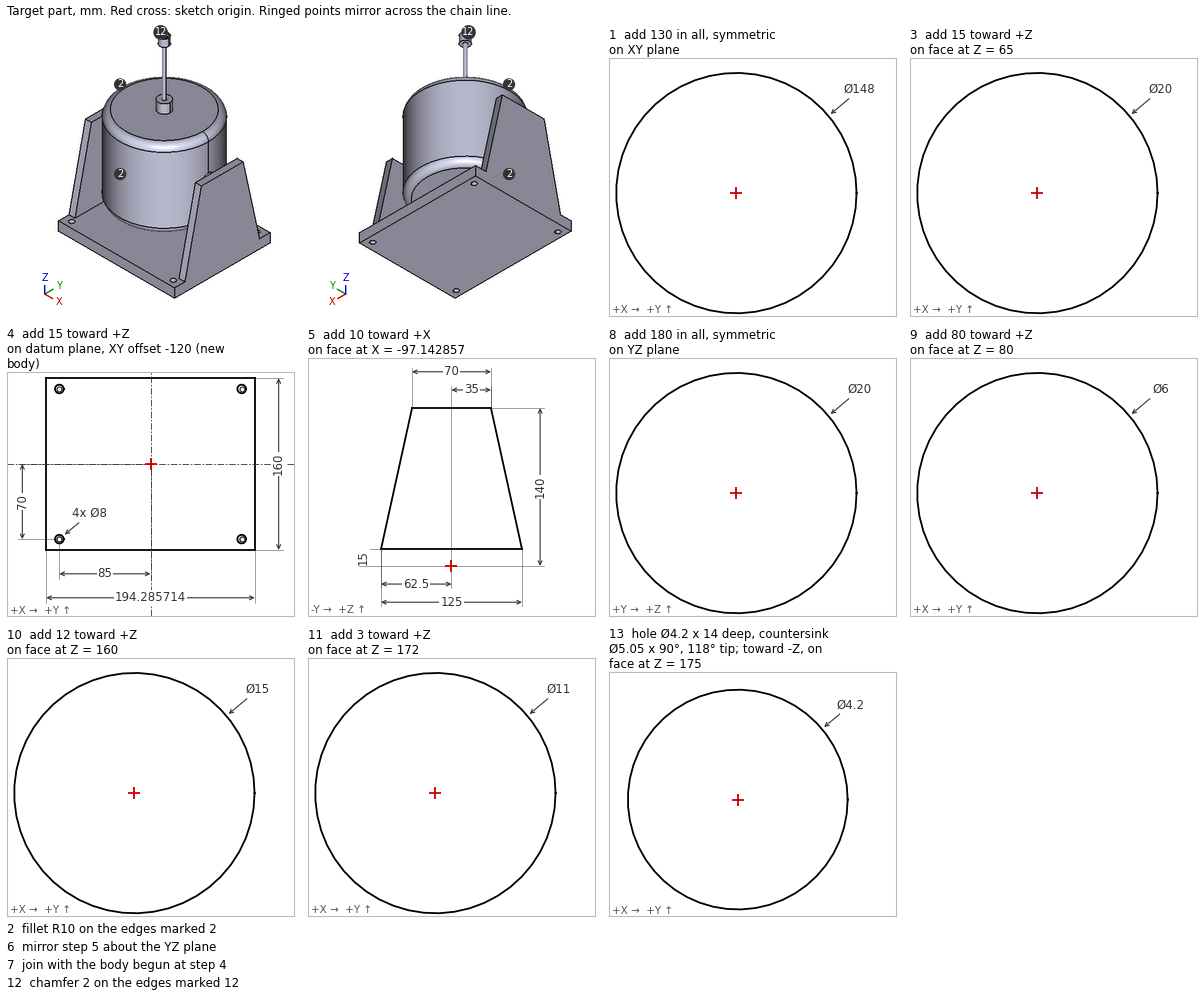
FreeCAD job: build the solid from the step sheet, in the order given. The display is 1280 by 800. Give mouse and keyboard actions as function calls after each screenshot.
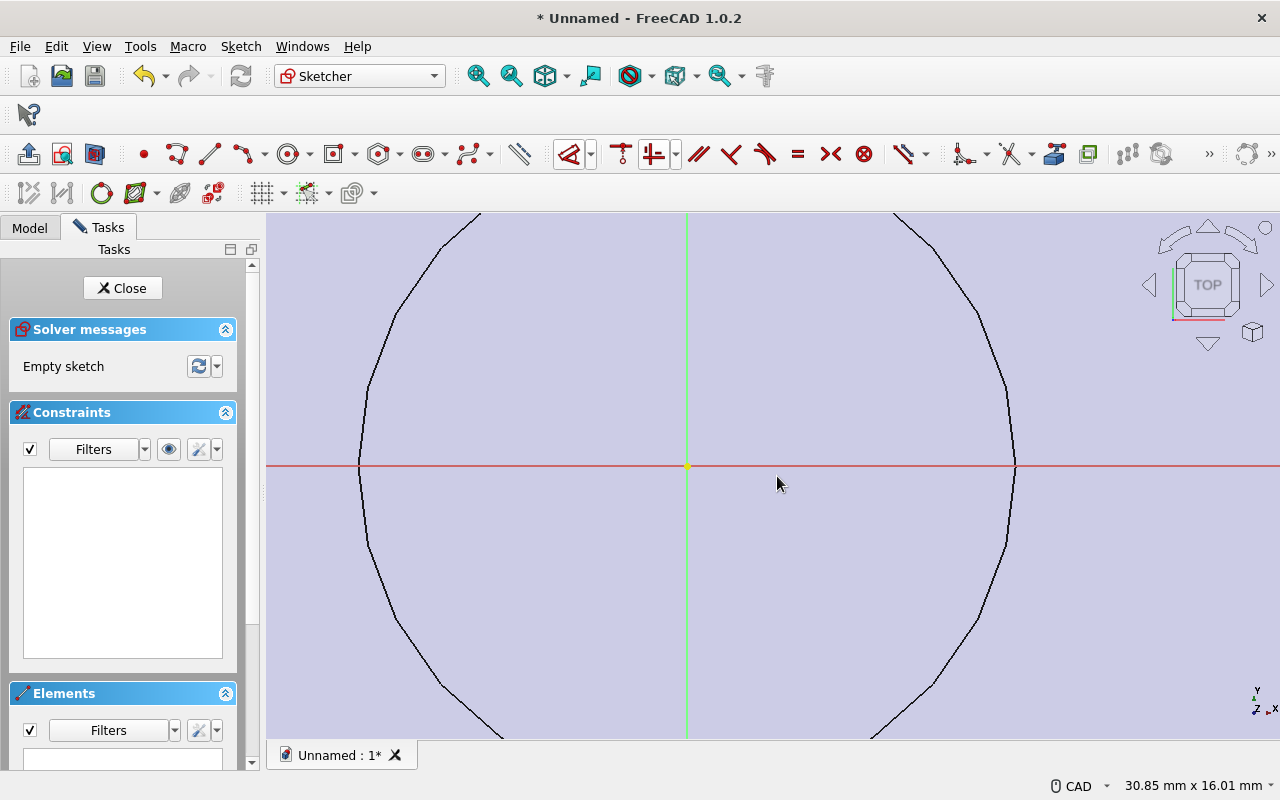
scroll(666, 455, up, 3)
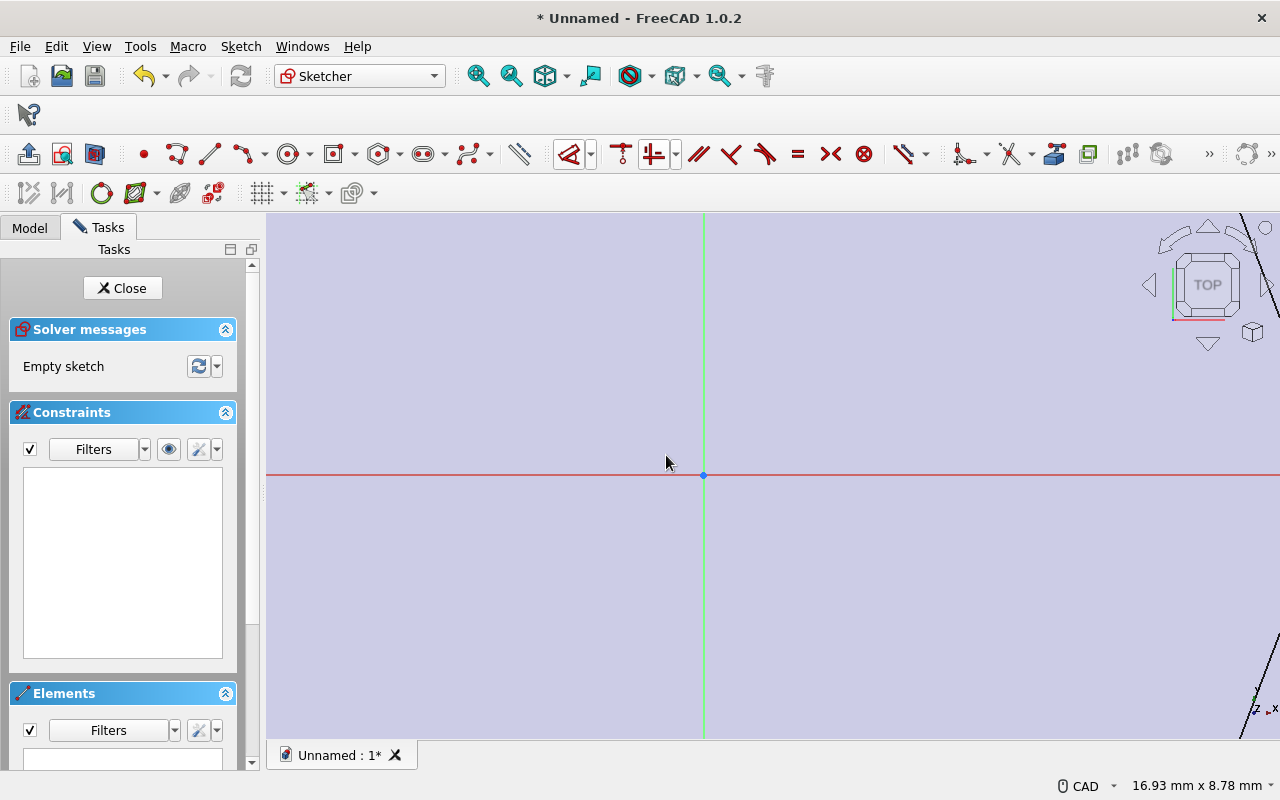
key(g)
key(c)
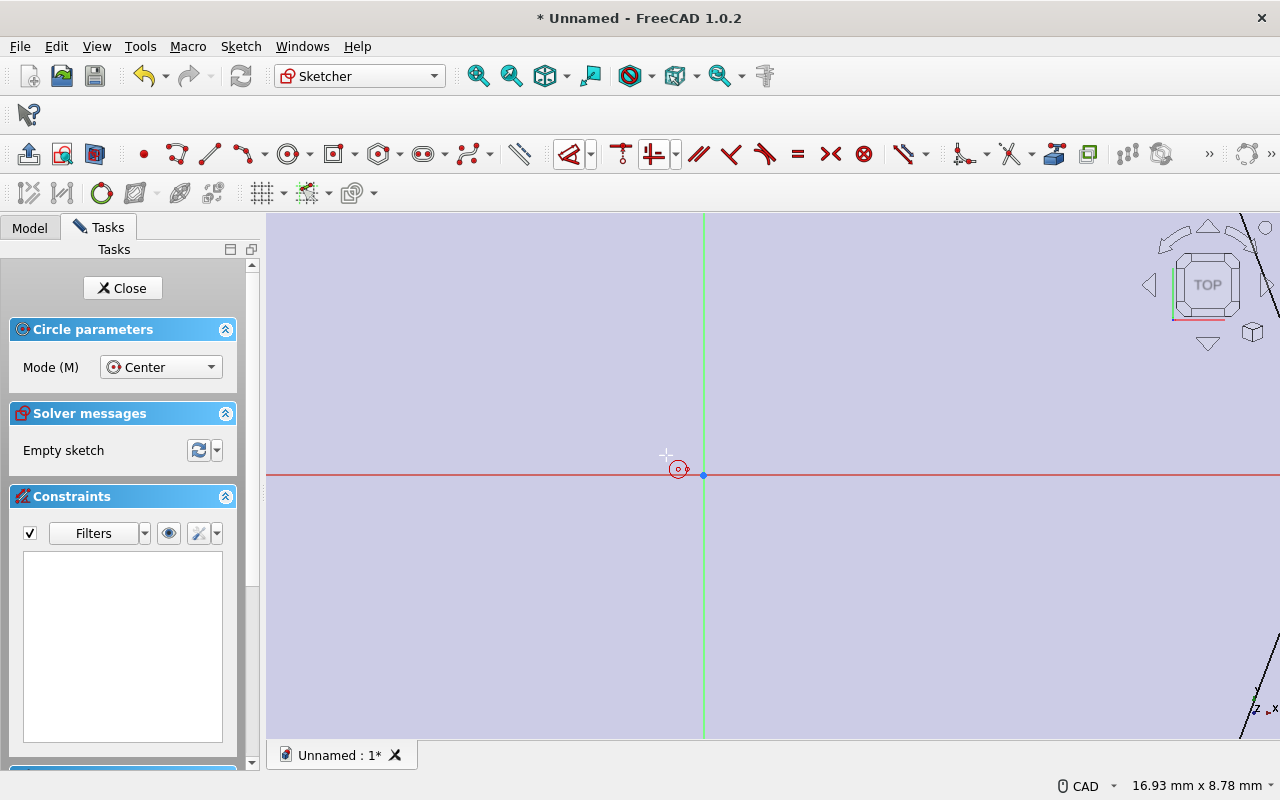
click(704, 475)
click(831, 348)
key(Escape)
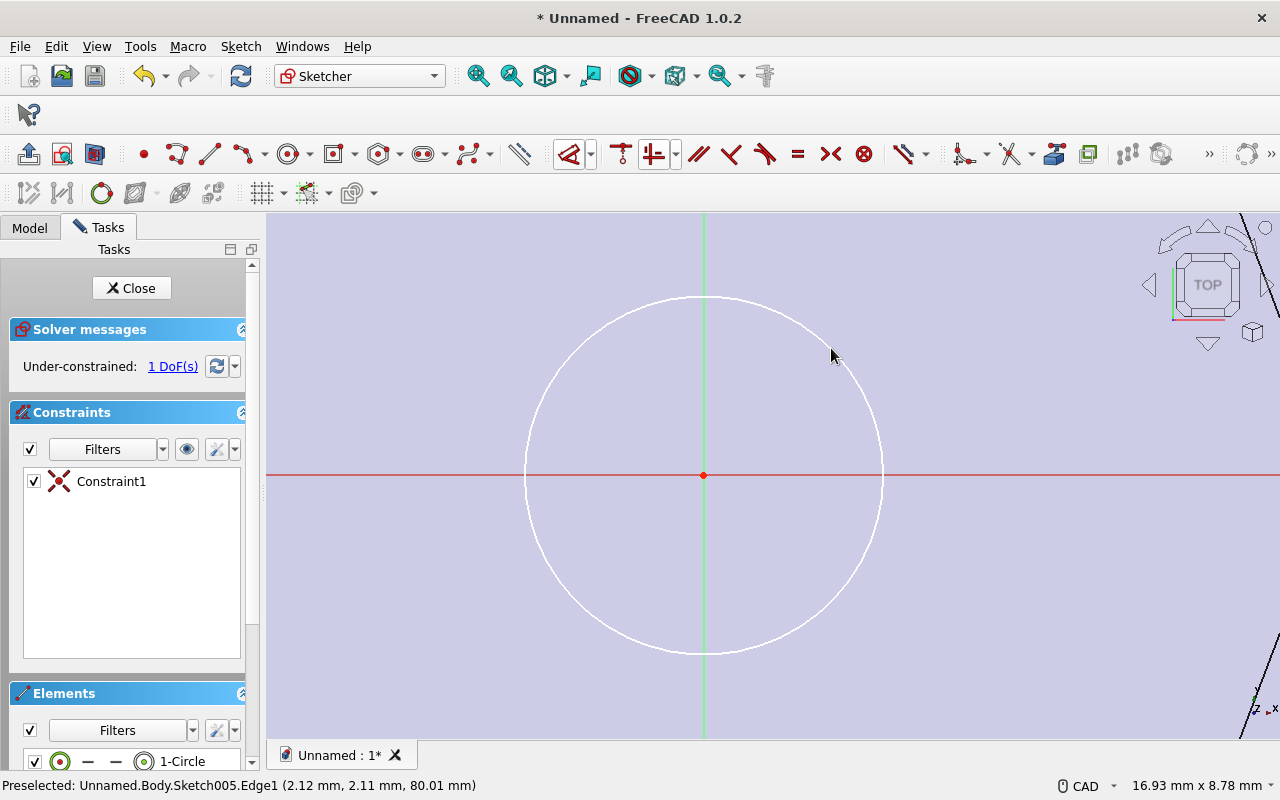
click(830, 348)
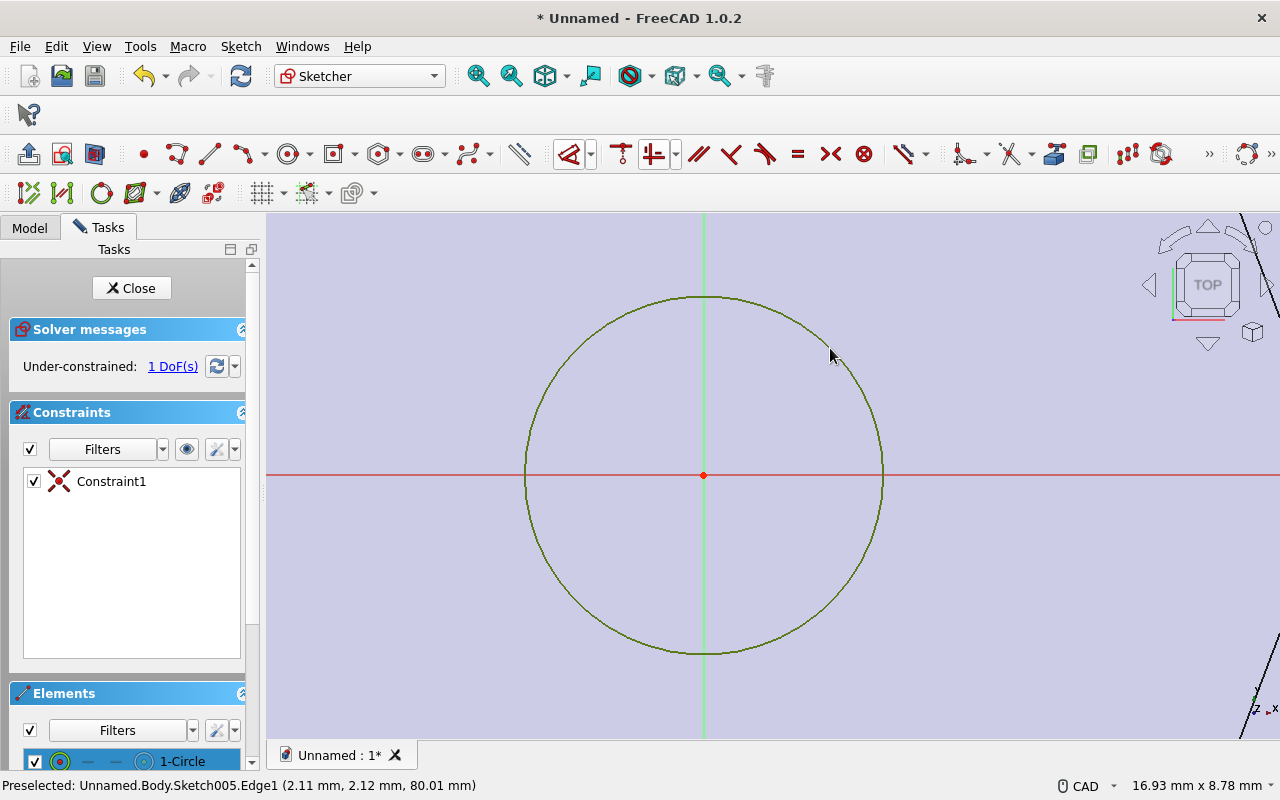
key(k)
key(o)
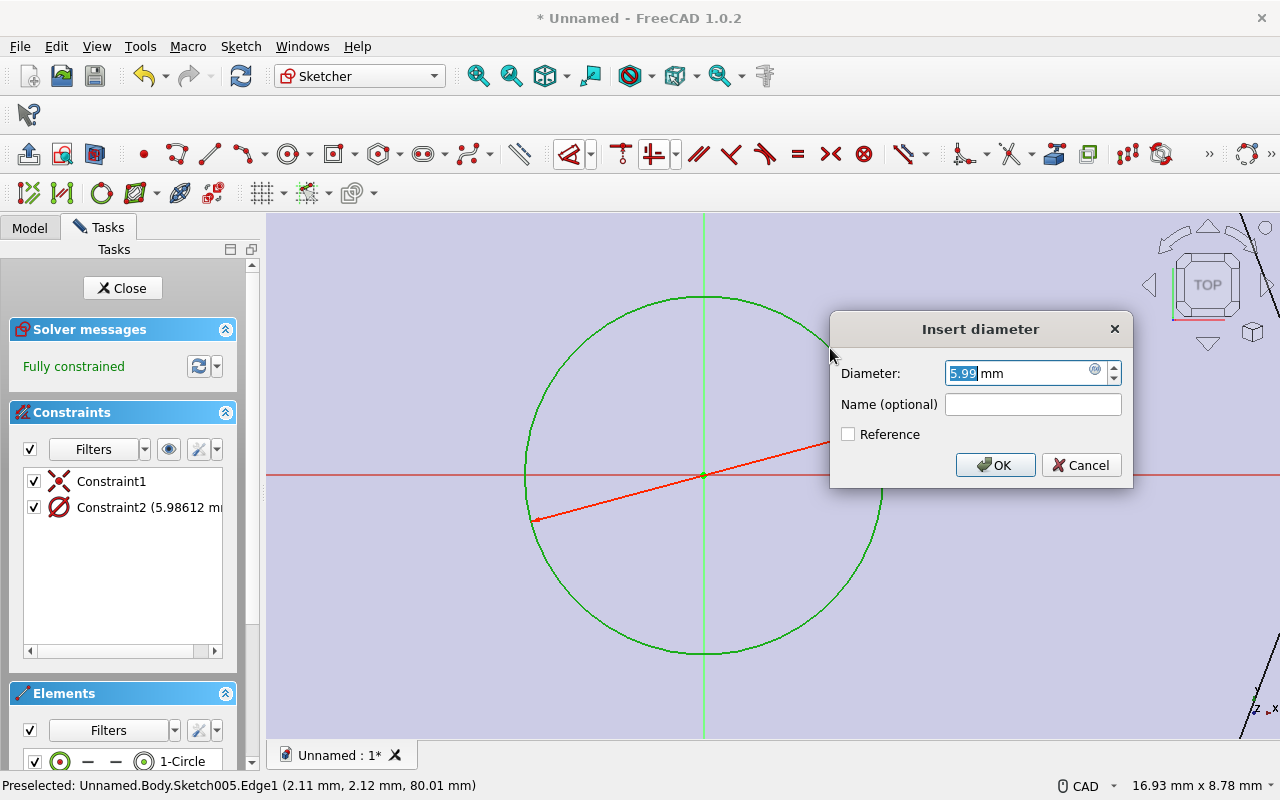
text(6)
key(Return)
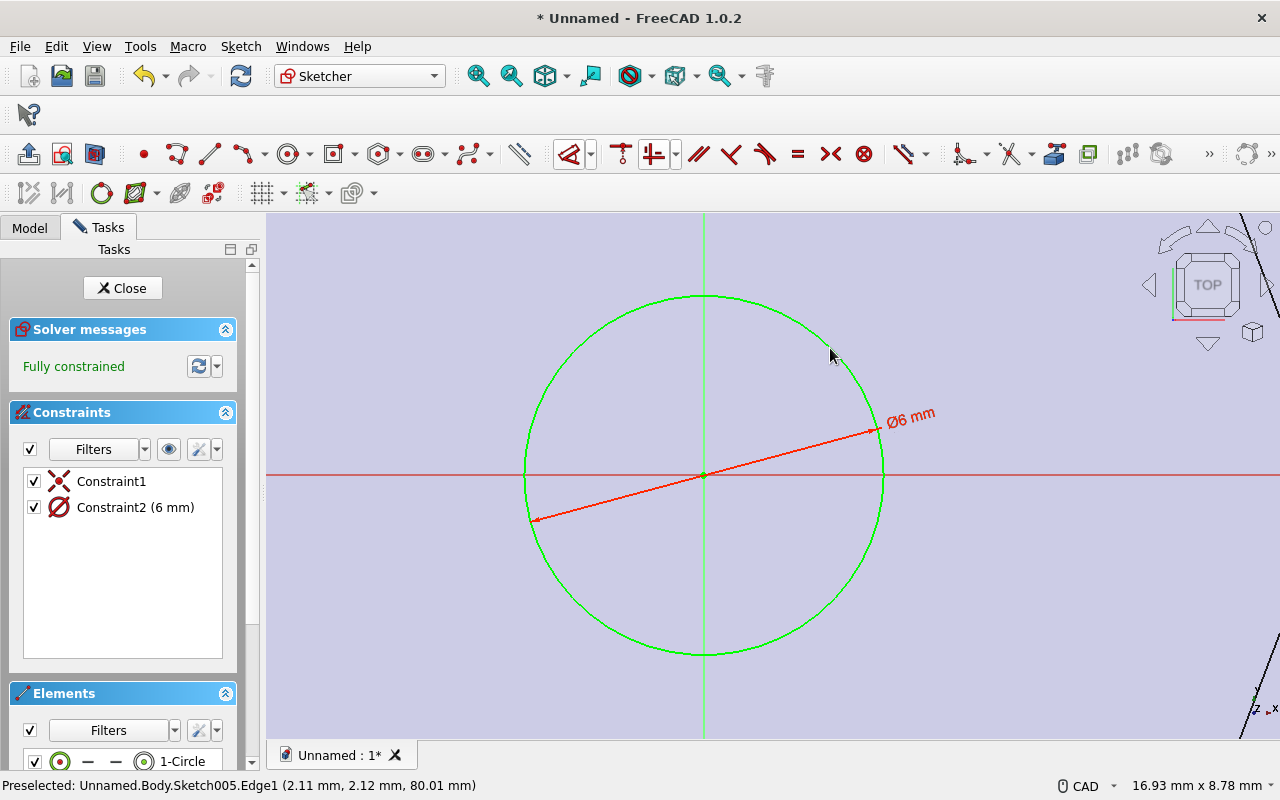
click(123, 288)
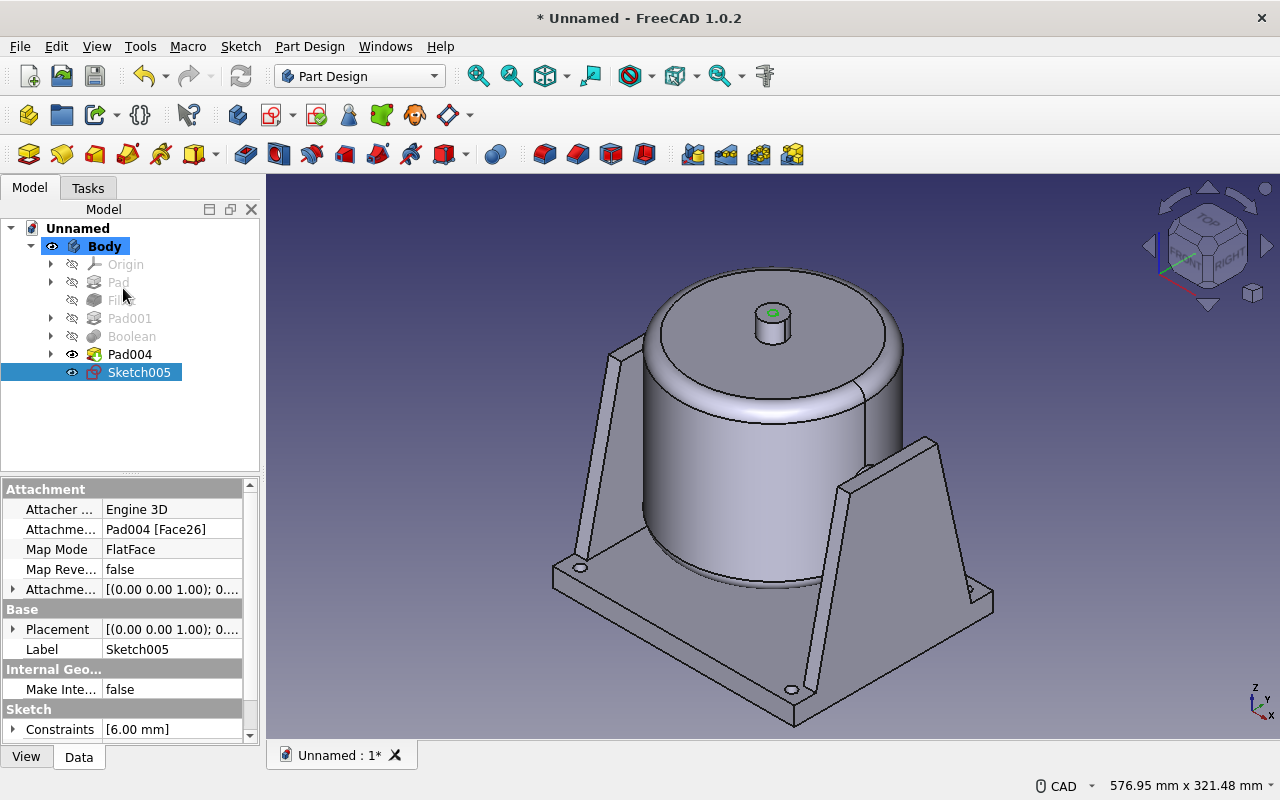
click(29, 154)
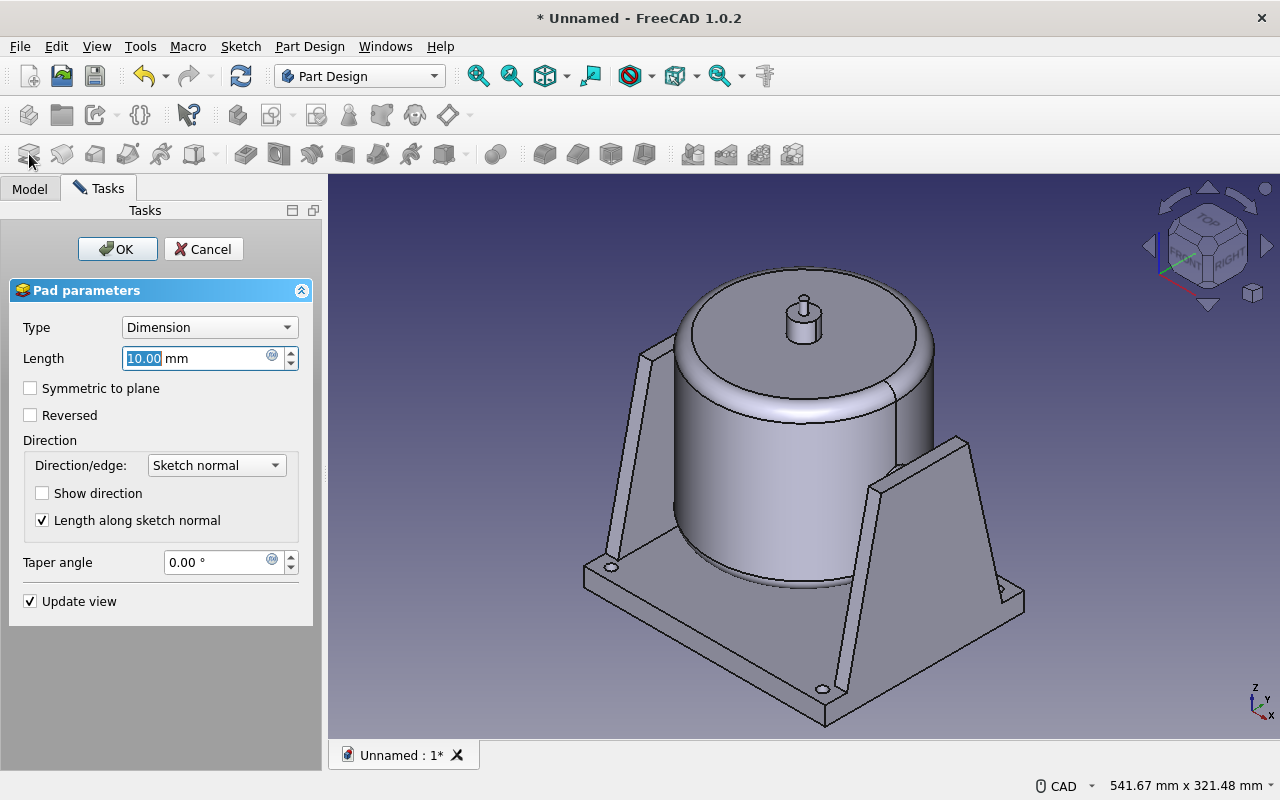
text(80)
key(Tab)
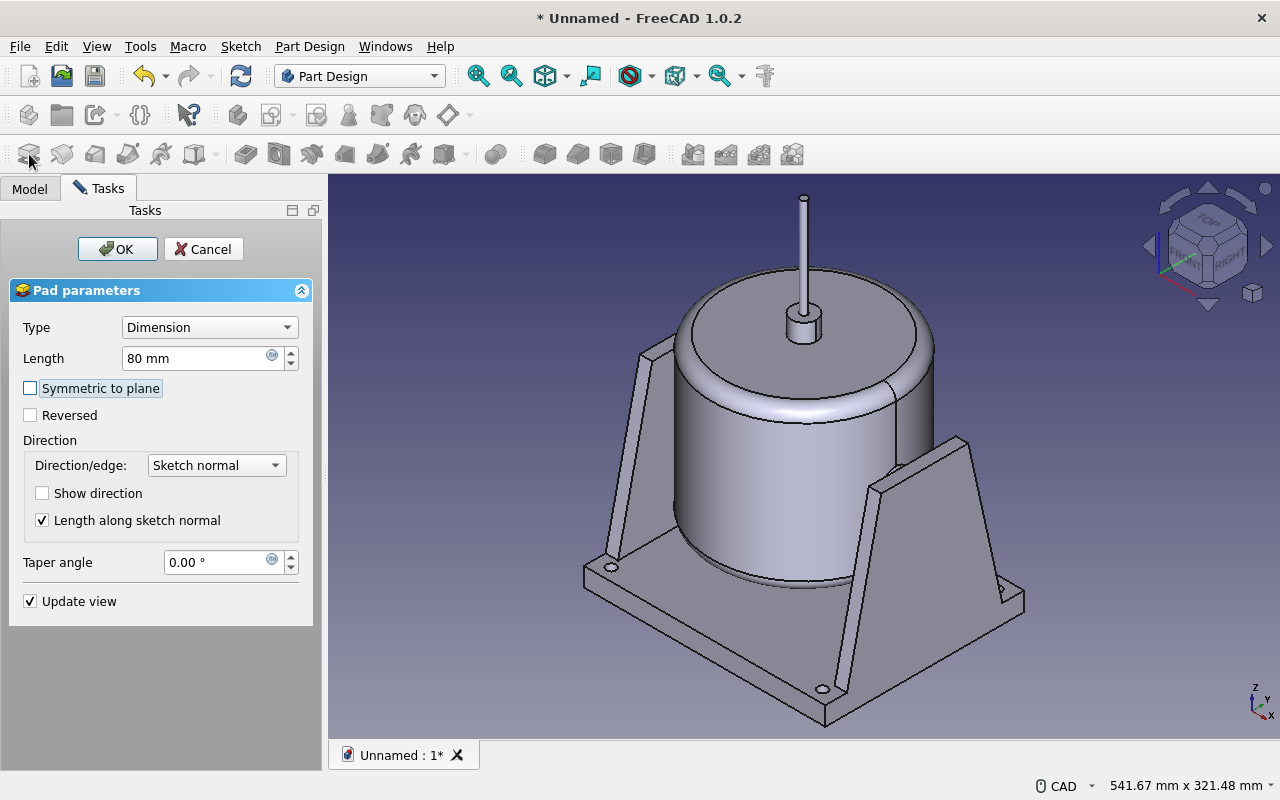
click(118, 249)